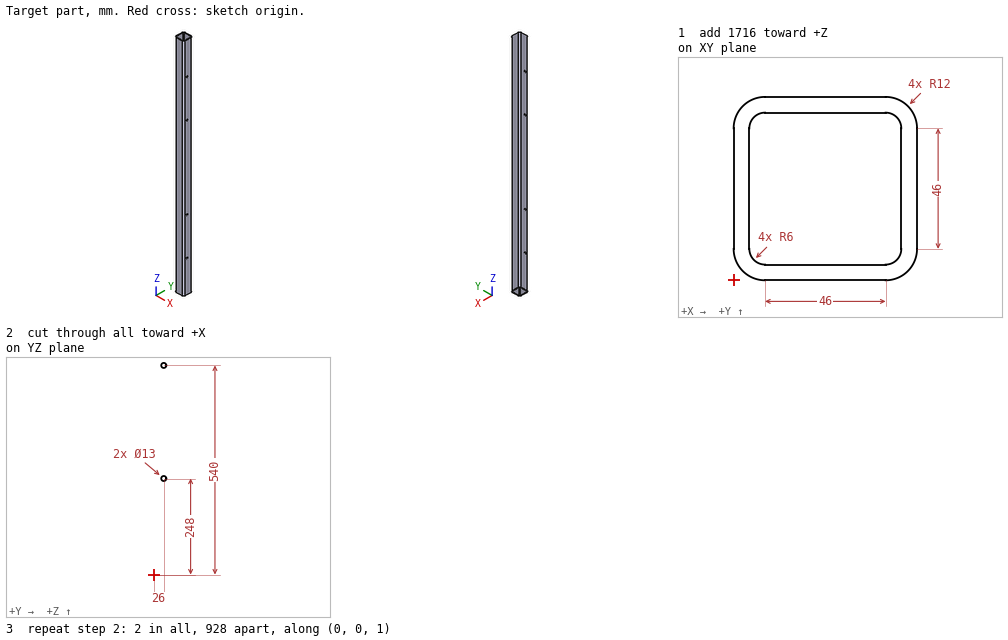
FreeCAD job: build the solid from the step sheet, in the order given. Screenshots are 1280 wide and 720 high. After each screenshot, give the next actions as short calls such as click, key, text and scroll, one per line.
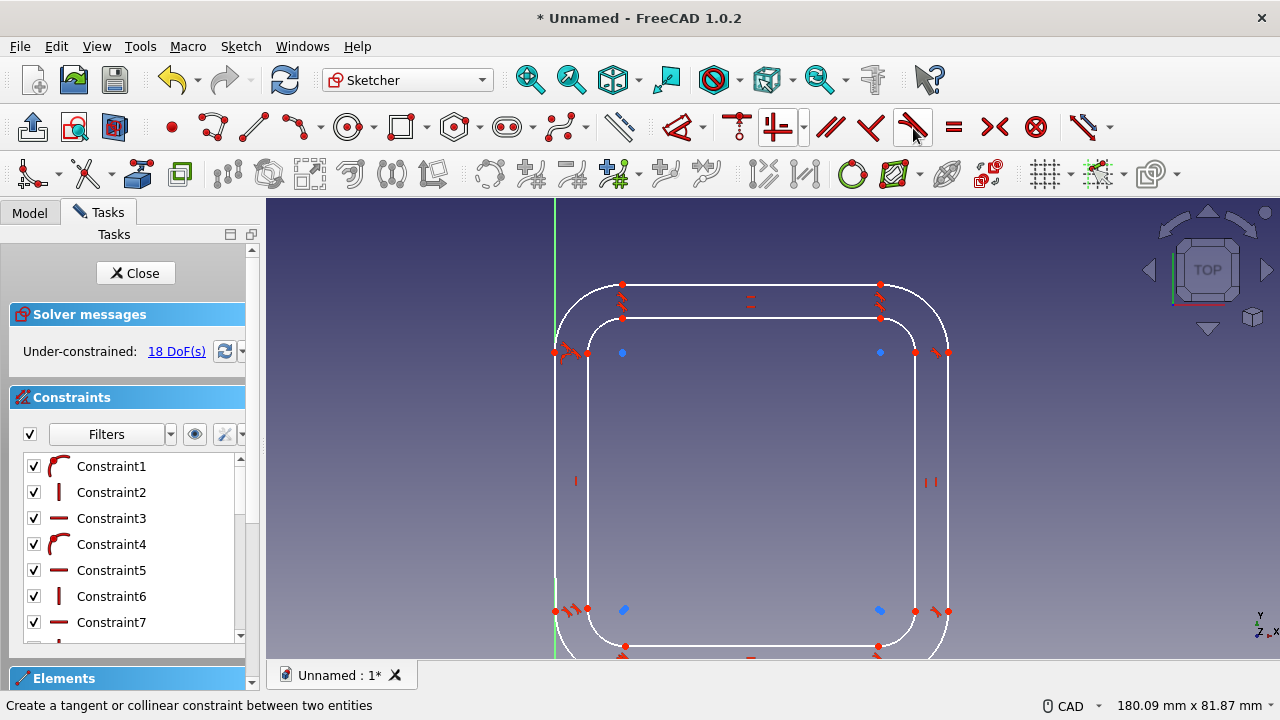
click(915, 430)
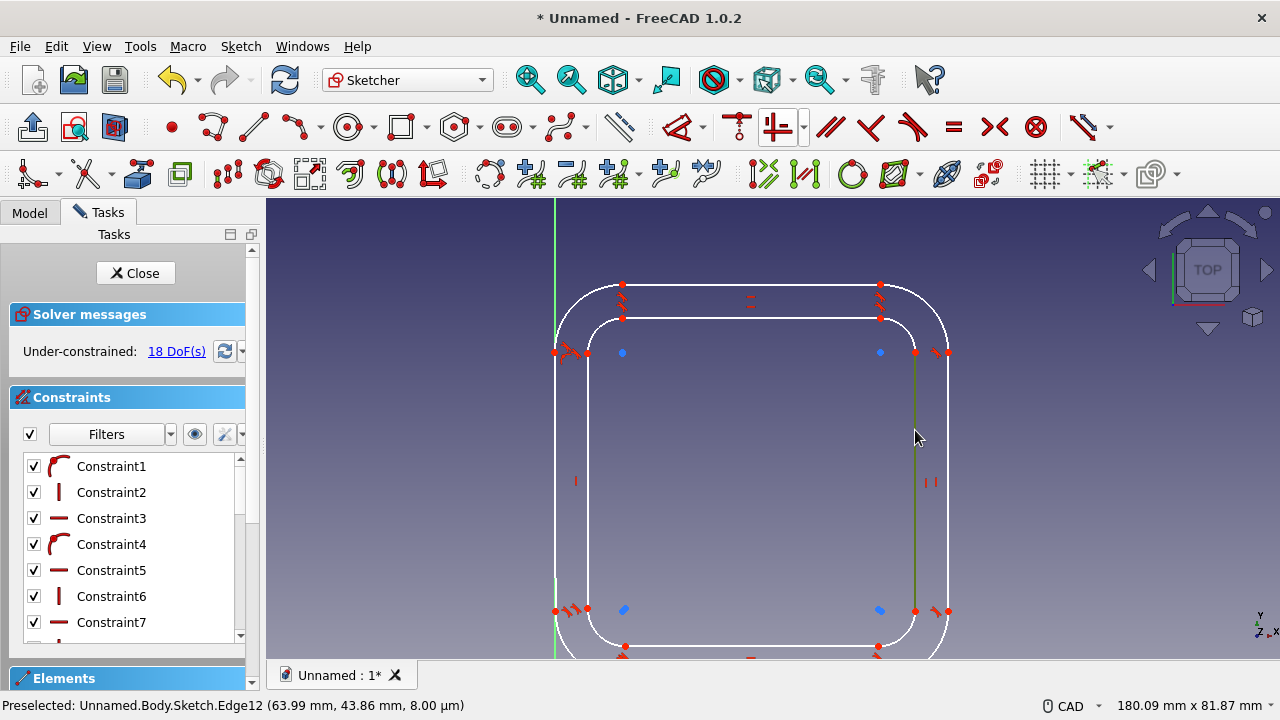
click(911, 337)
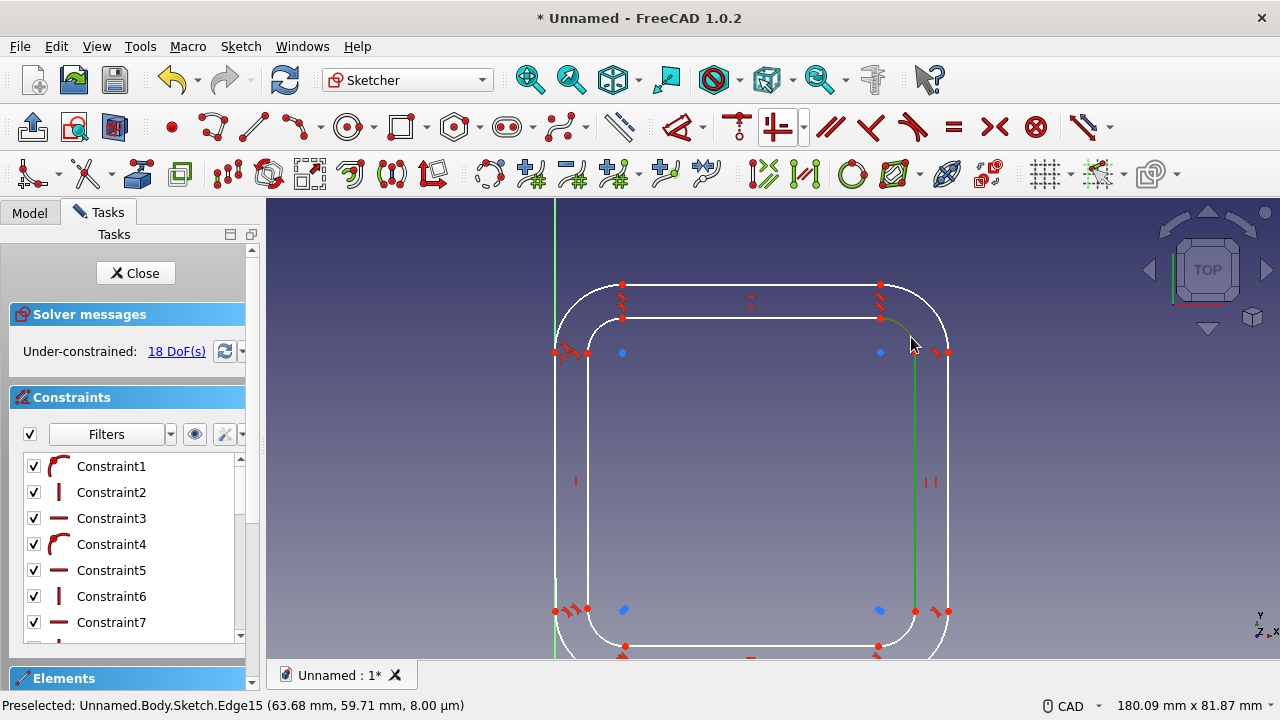
click(913, 128)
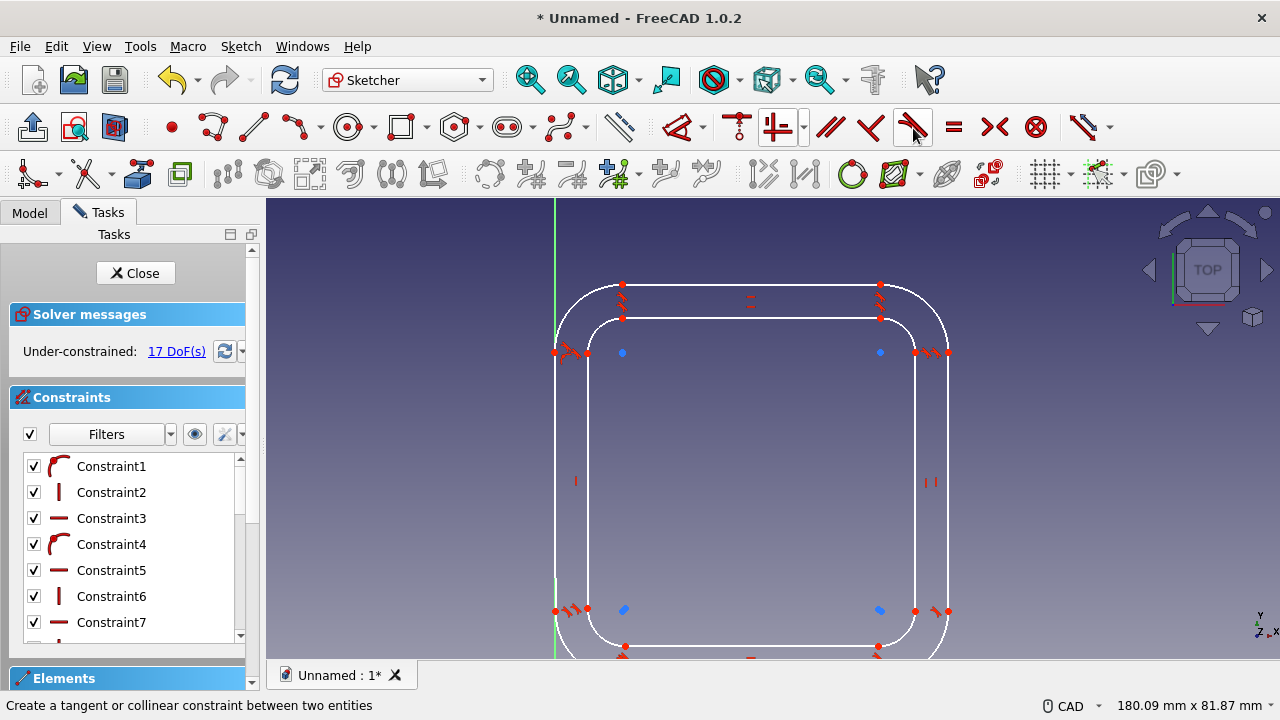
click(915, 430)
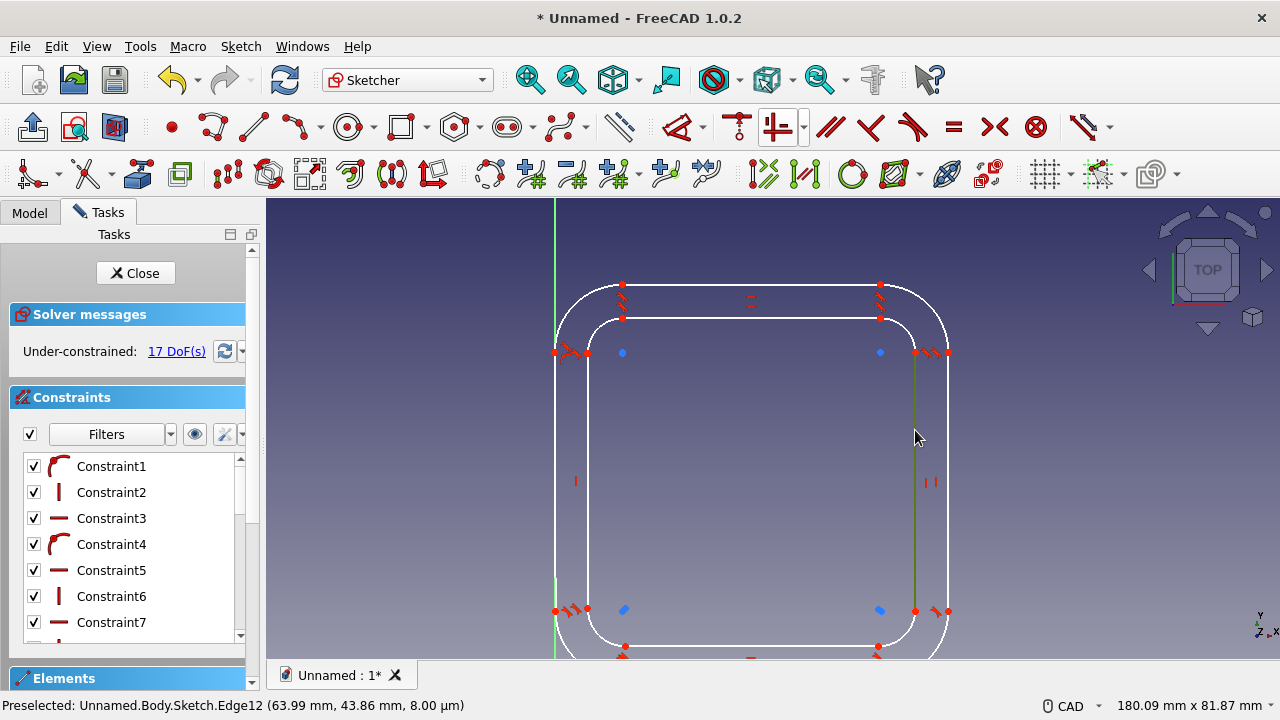
click(910, 628)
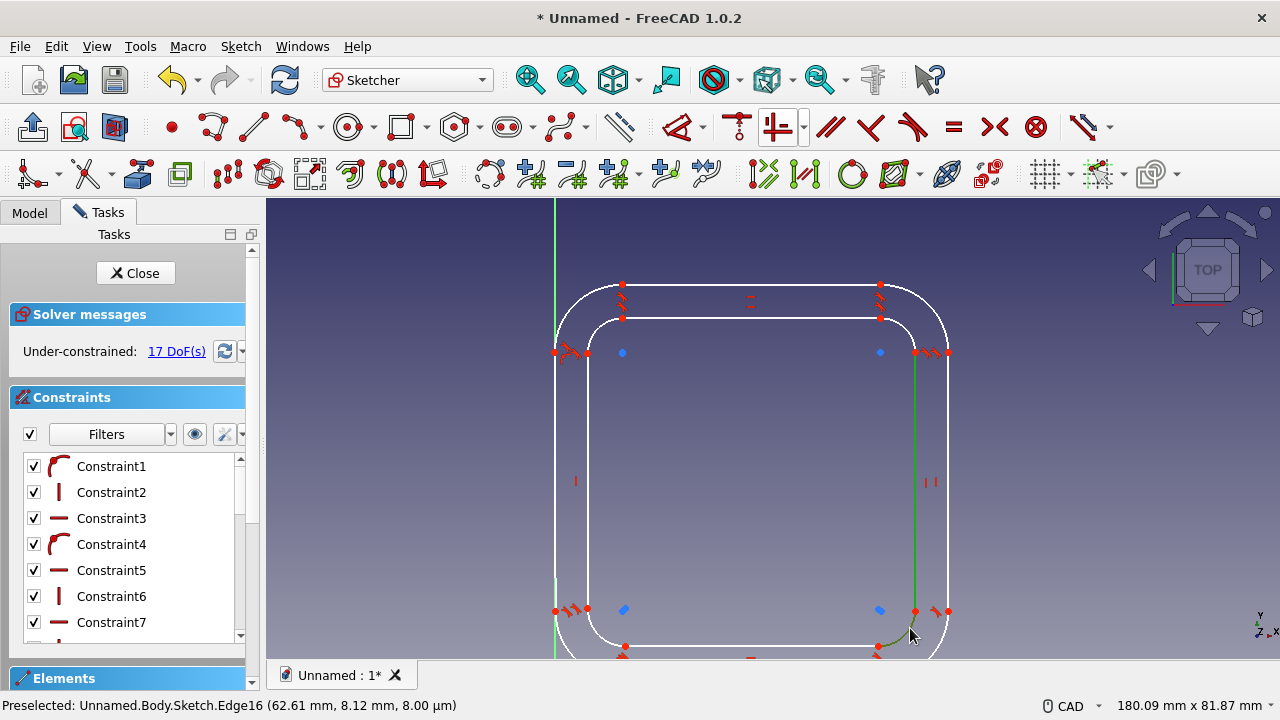
click(913, 128)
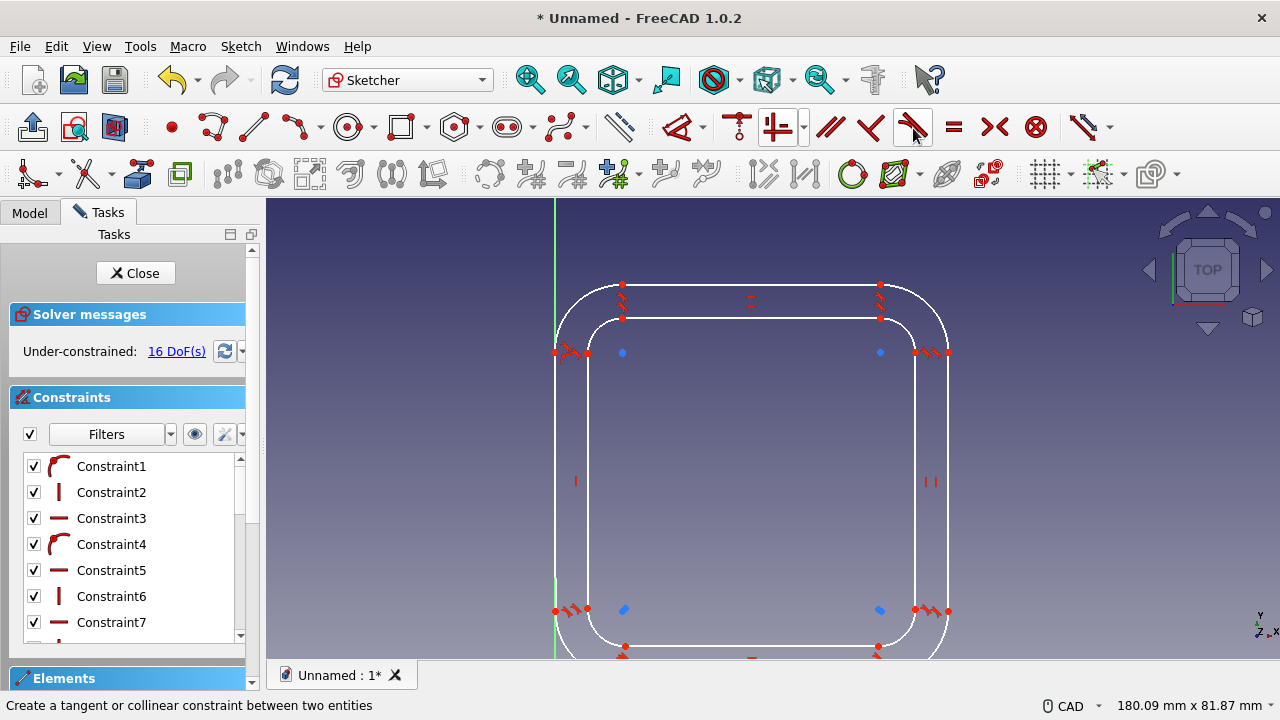
scroll(608, 322, down, 2)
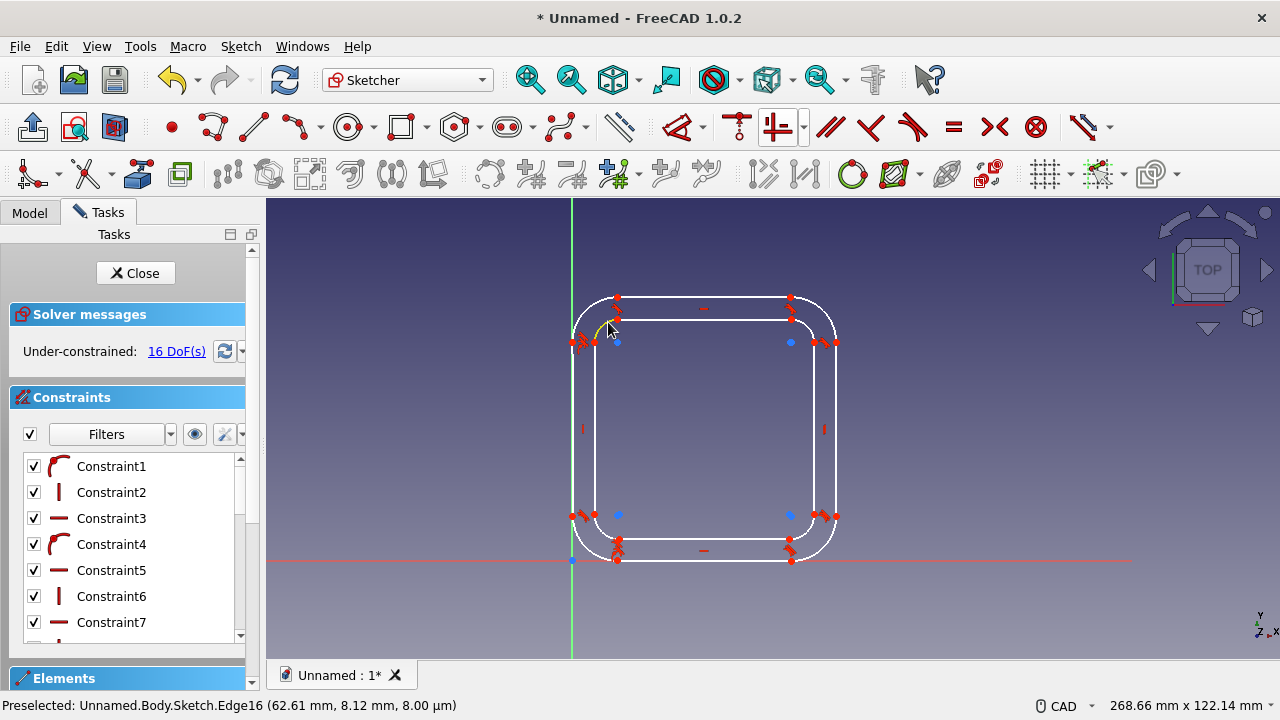
click(670, 561)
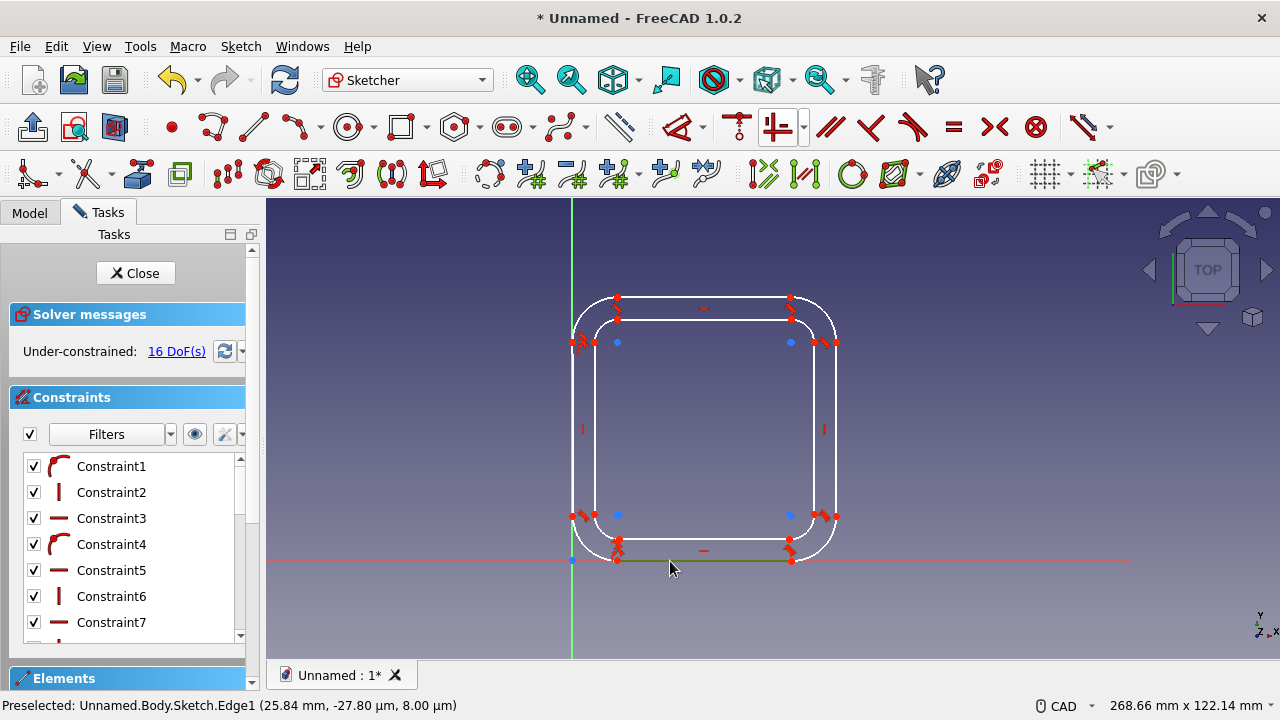
key(h)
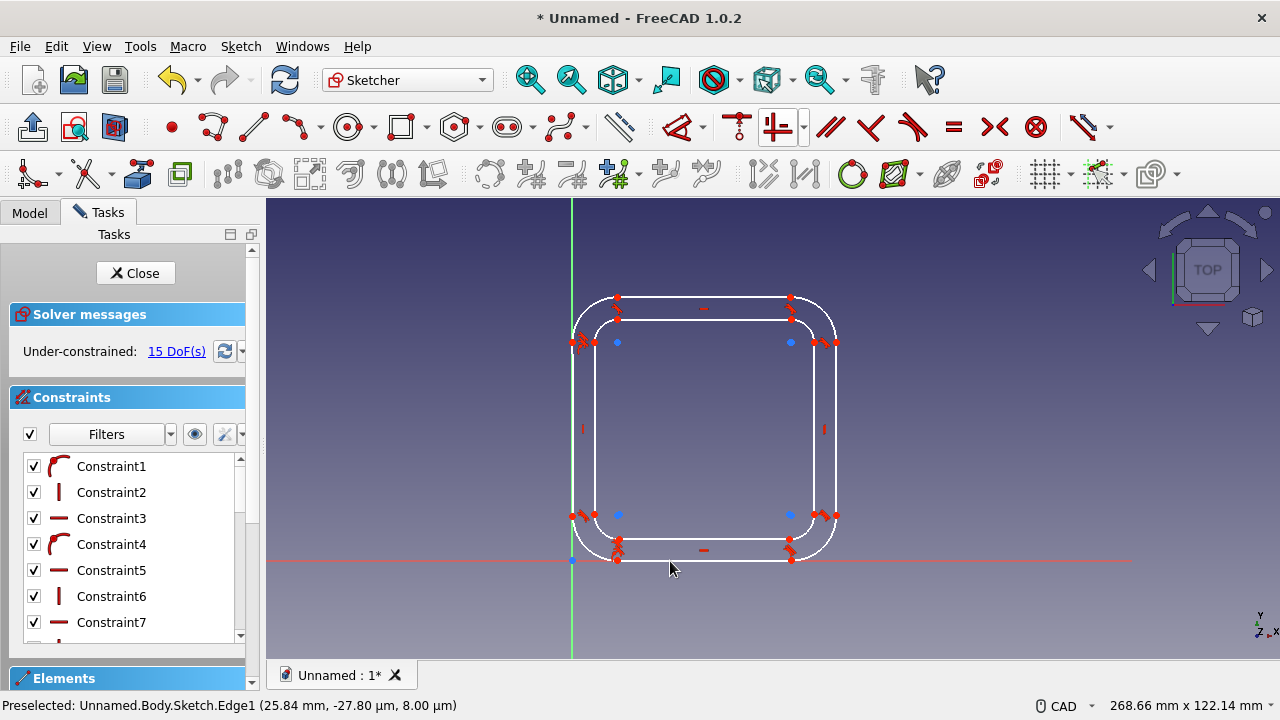
click(573, 395)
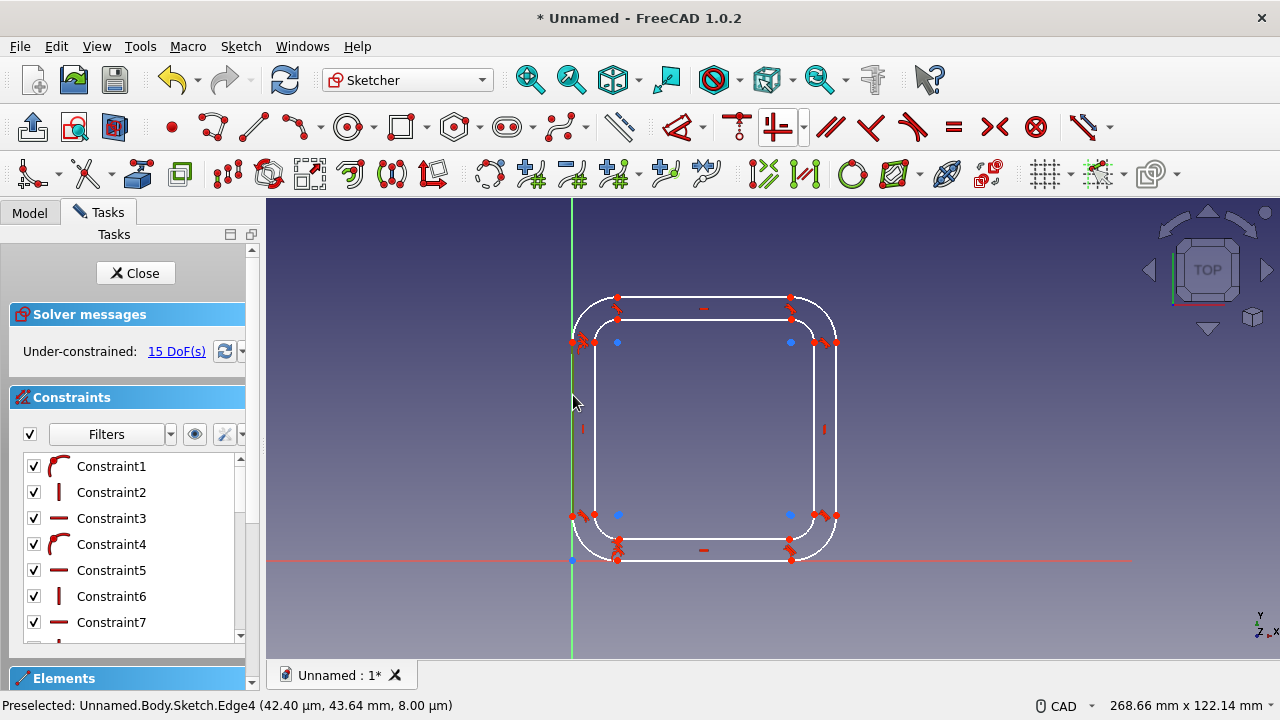
click(804, 128)